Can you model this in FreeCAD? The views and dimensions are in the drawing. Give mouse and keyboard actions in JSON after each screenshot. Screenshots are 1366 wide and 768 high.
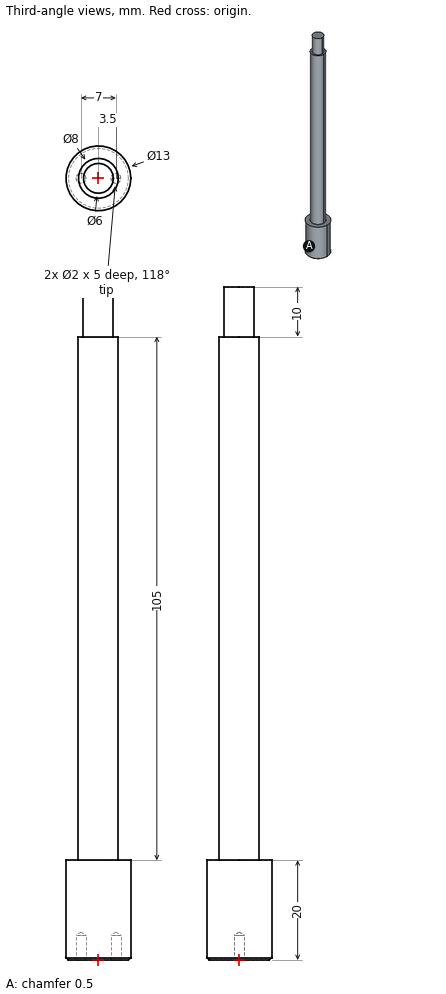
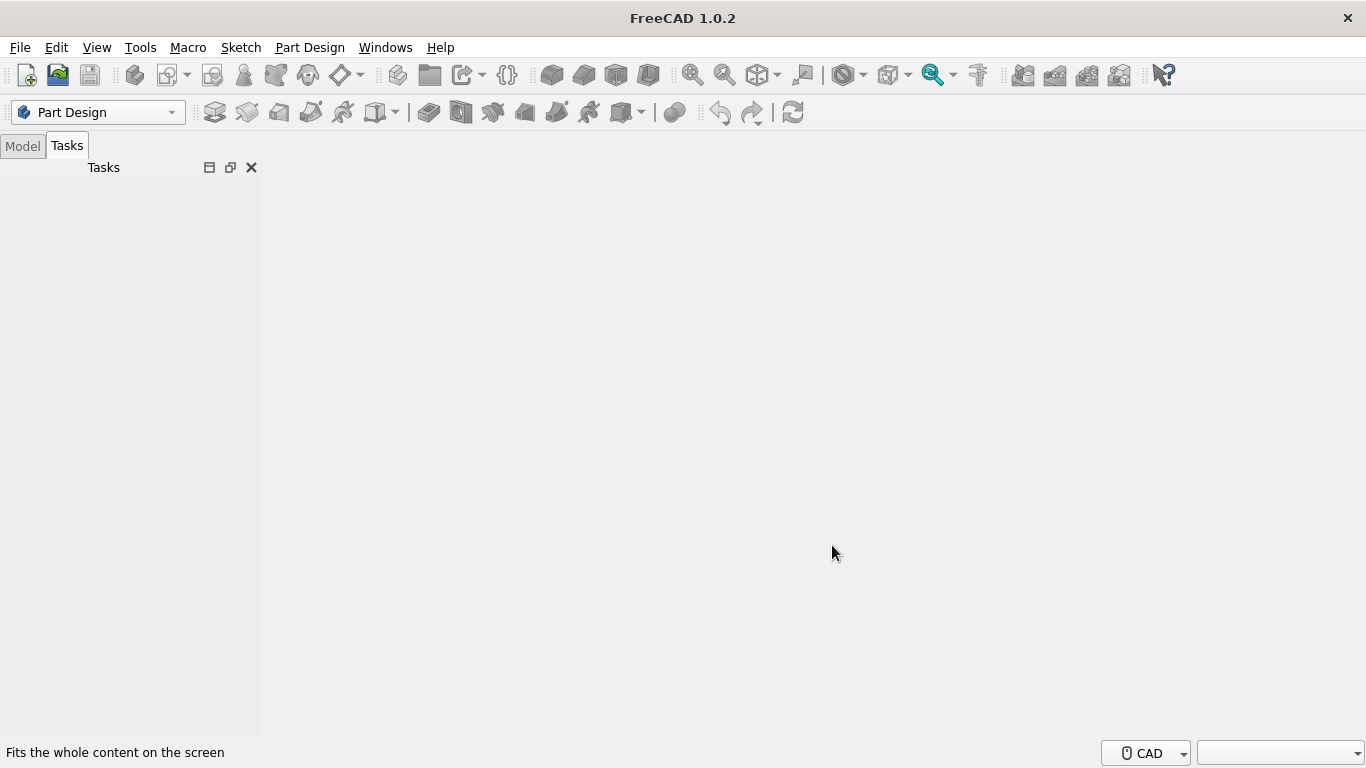
{"action": "key", "text": "ctrl+n"}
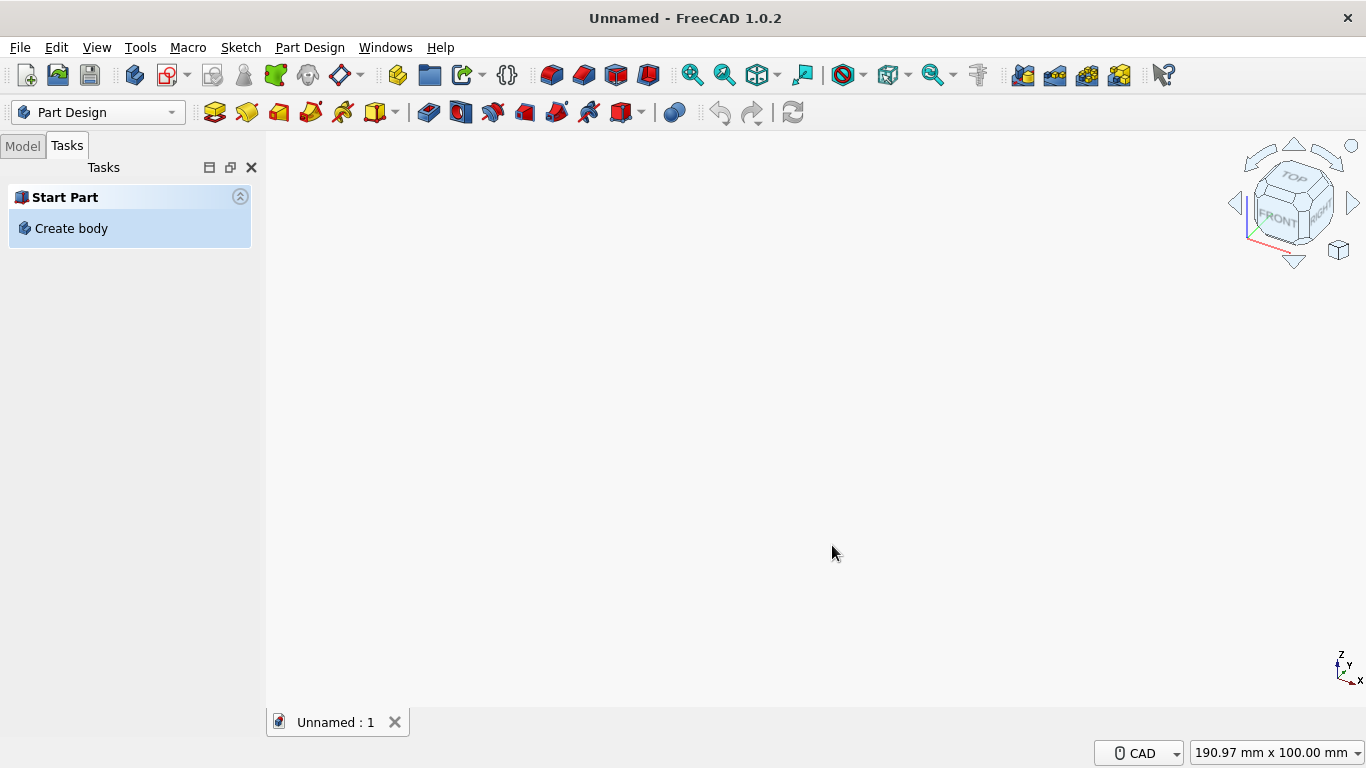
{"action": "left_click", "coordinate": [168, 76]}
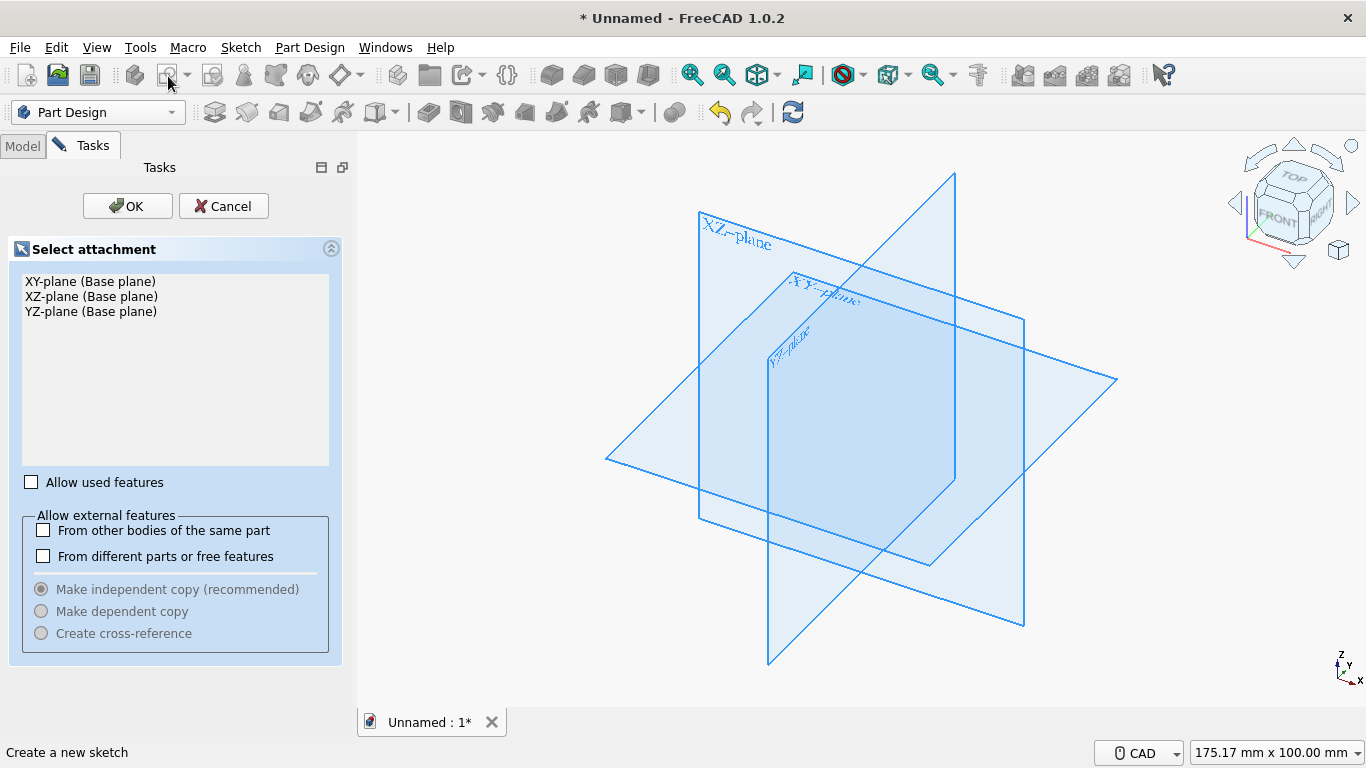
{"action": "left_click", "coordinate": [82, 282]}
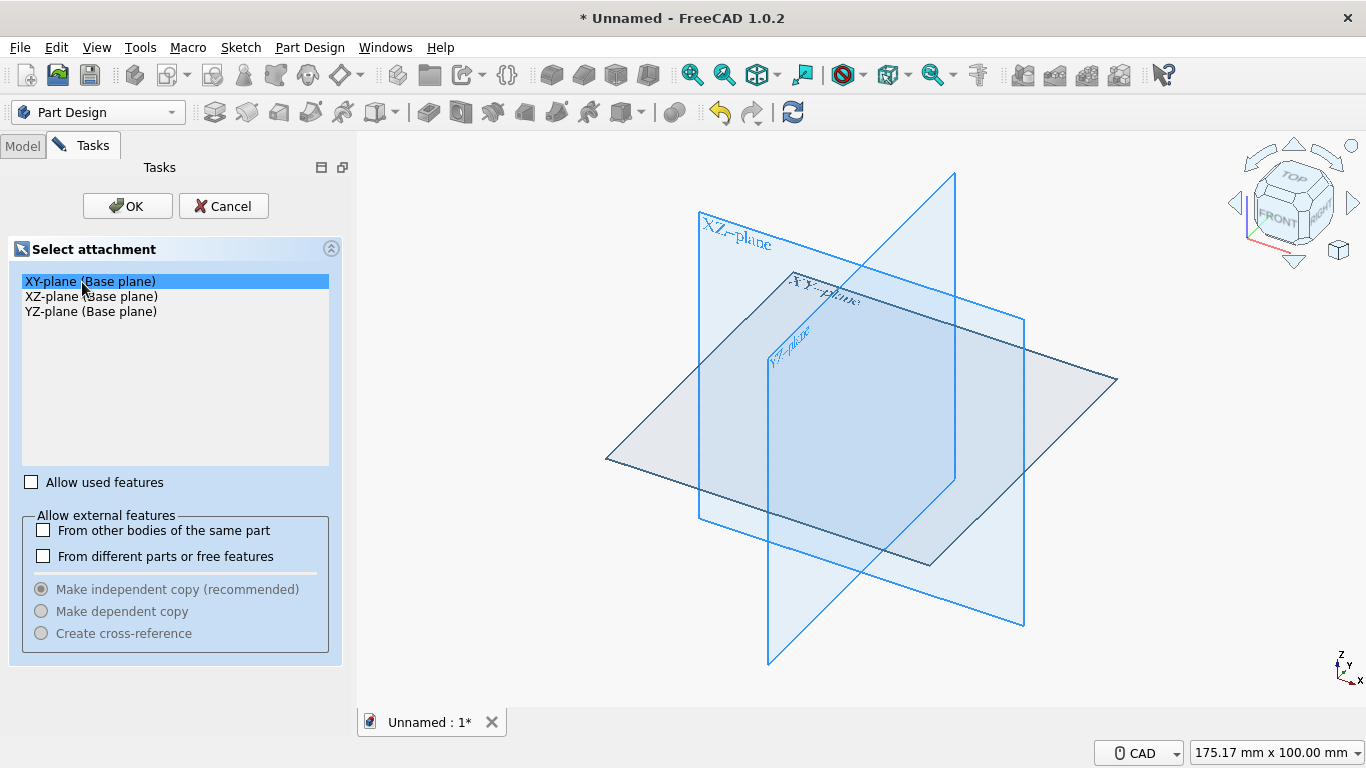
{"action": "left_click", "coordinate": [128, 206]}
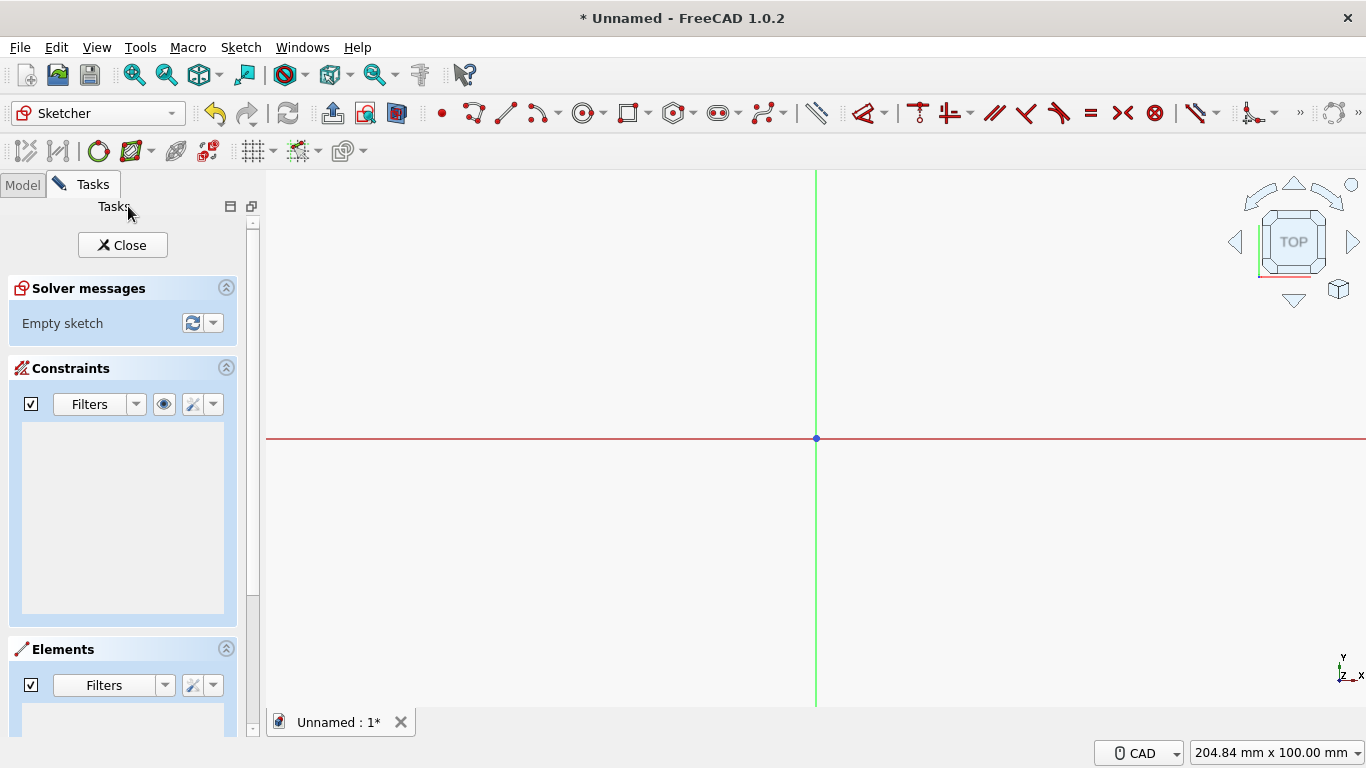
{"action": "scroll", "coordinate": [833, 438], "scroll_direction": "up", "scroll_amount": 8}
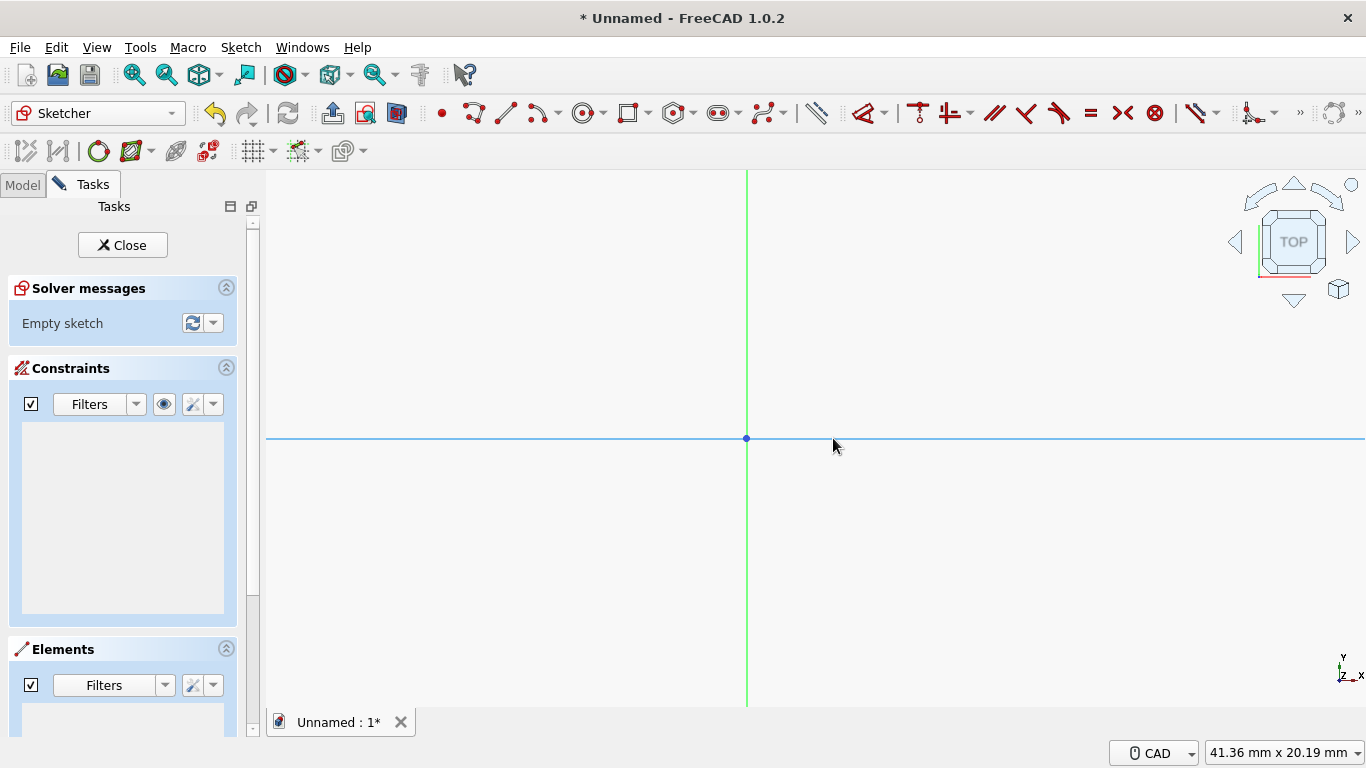
{"action": "key", "text": "g c"}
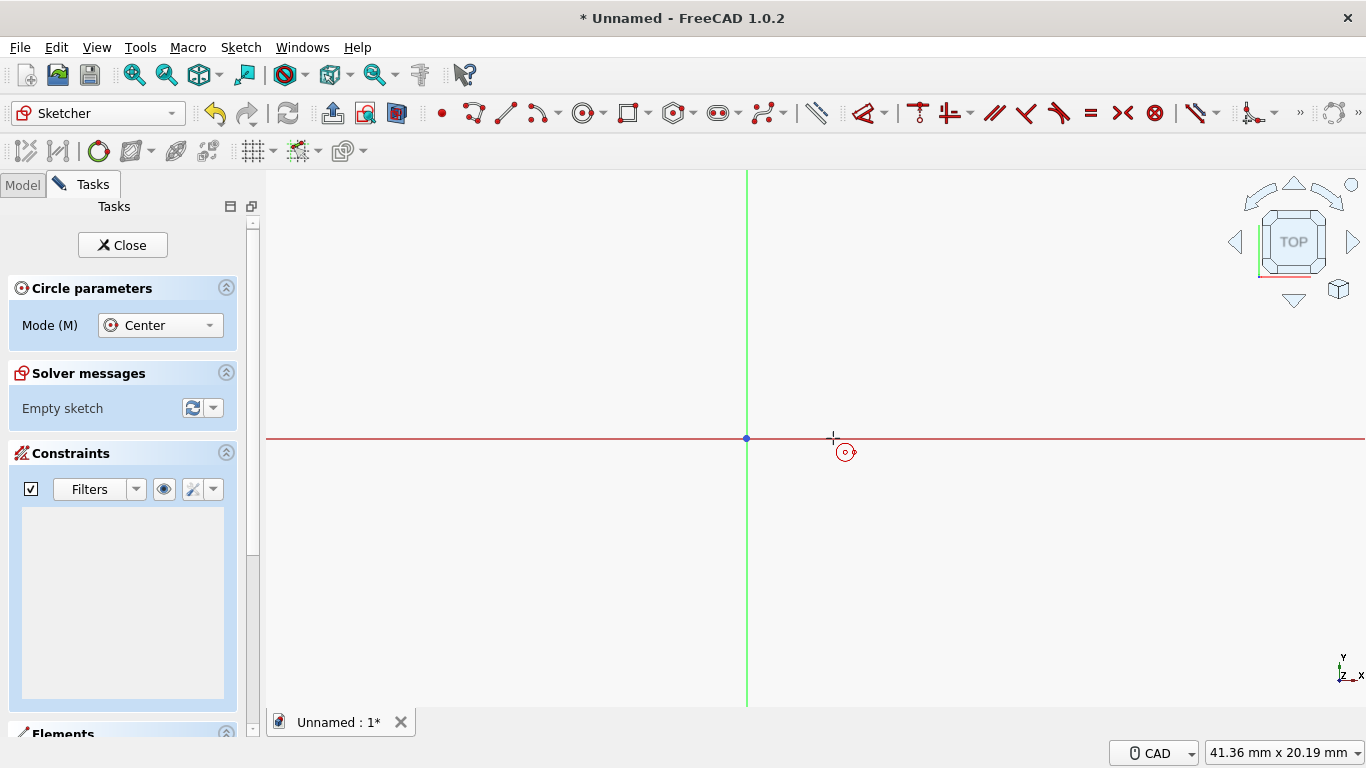
{"action": "left_click", "coordinate": [747, 438]}
{"action": "left_click", "coordinate": [869, 316]}
{"action": "key", "text": "Escape"}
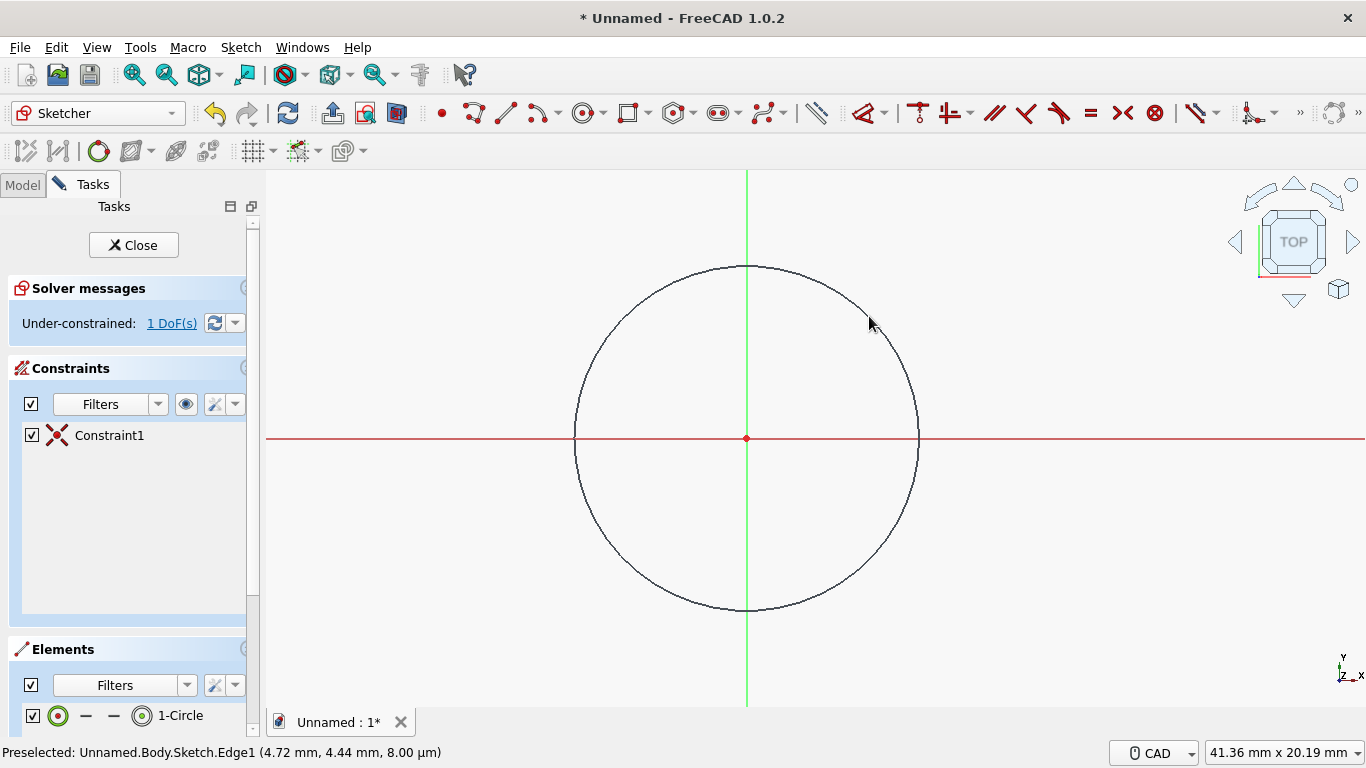
{"action": "left_click", "coordinate": [868, 316]}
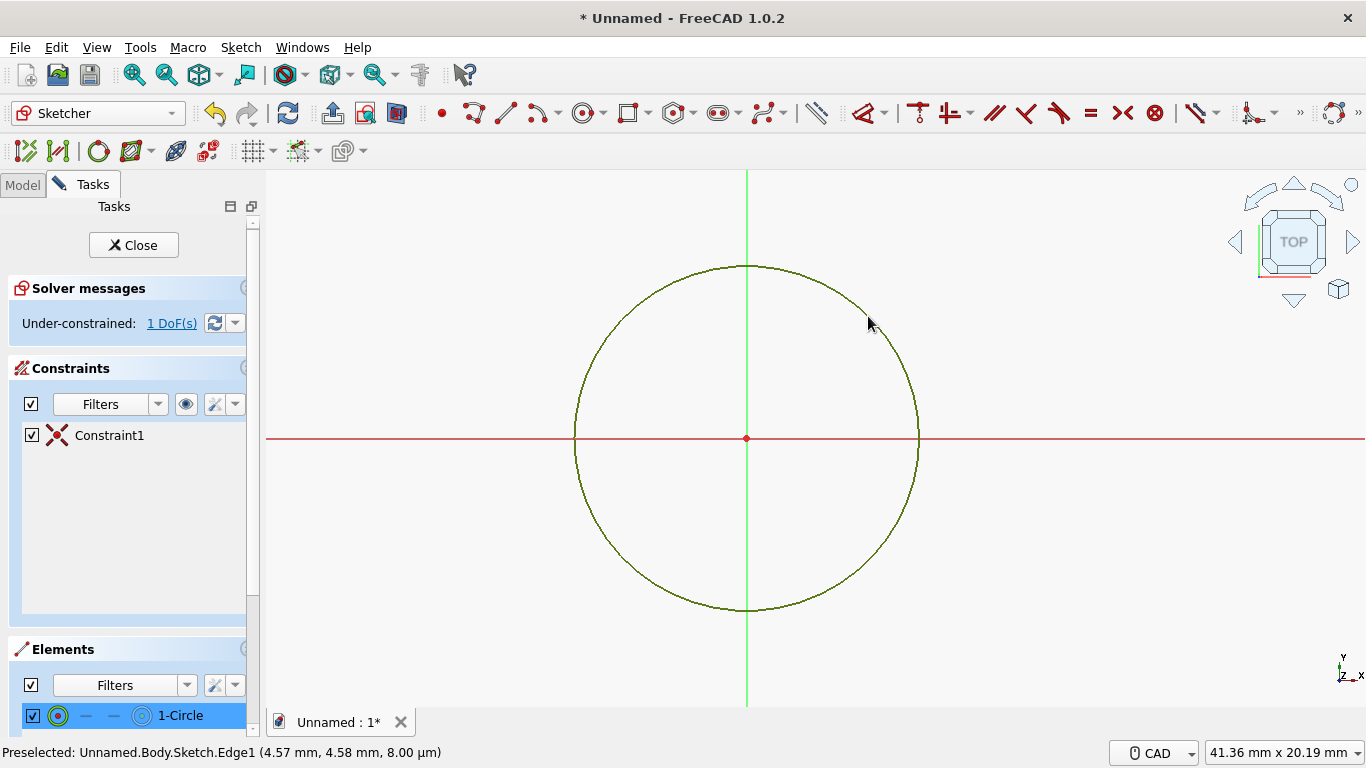
{"action": "key", "text": "k o"}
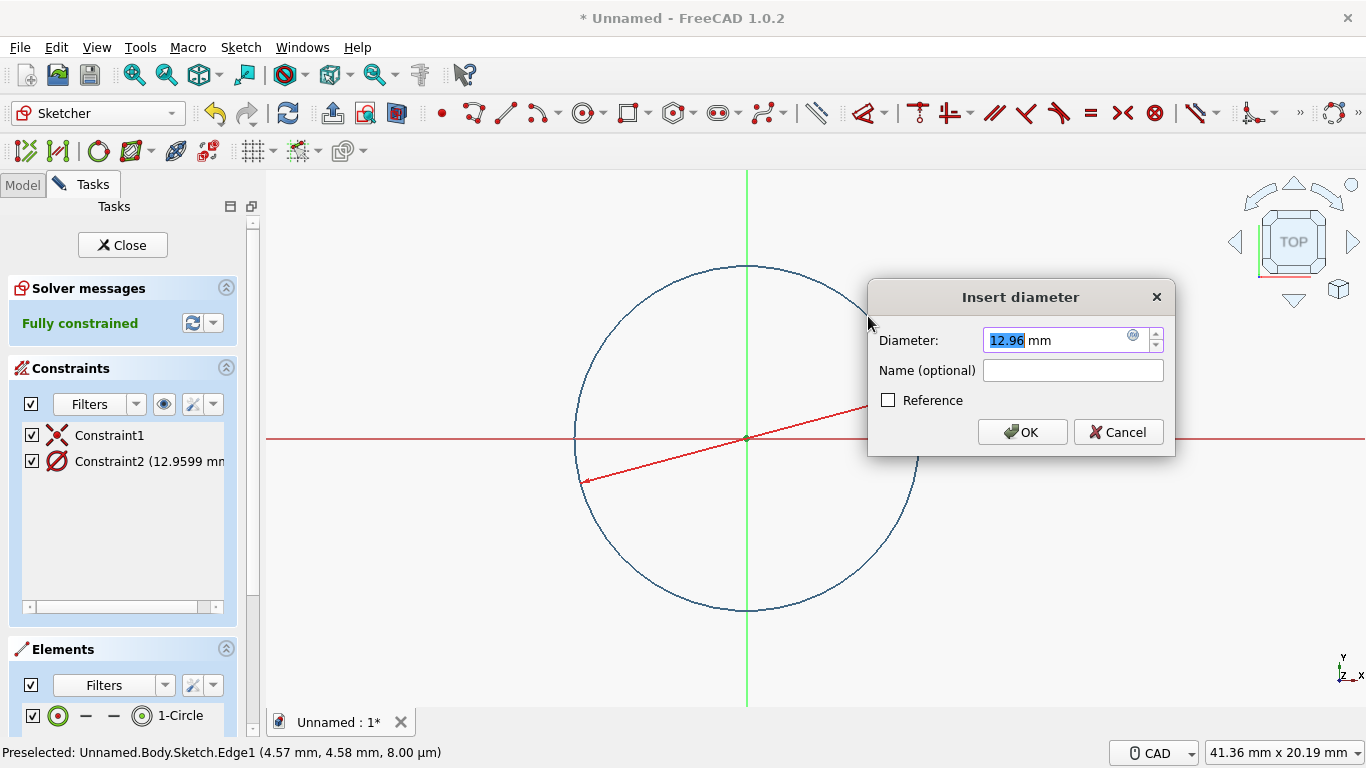
{"action": "type", "text": "13"}
{"action": "key", "text": "Return"}